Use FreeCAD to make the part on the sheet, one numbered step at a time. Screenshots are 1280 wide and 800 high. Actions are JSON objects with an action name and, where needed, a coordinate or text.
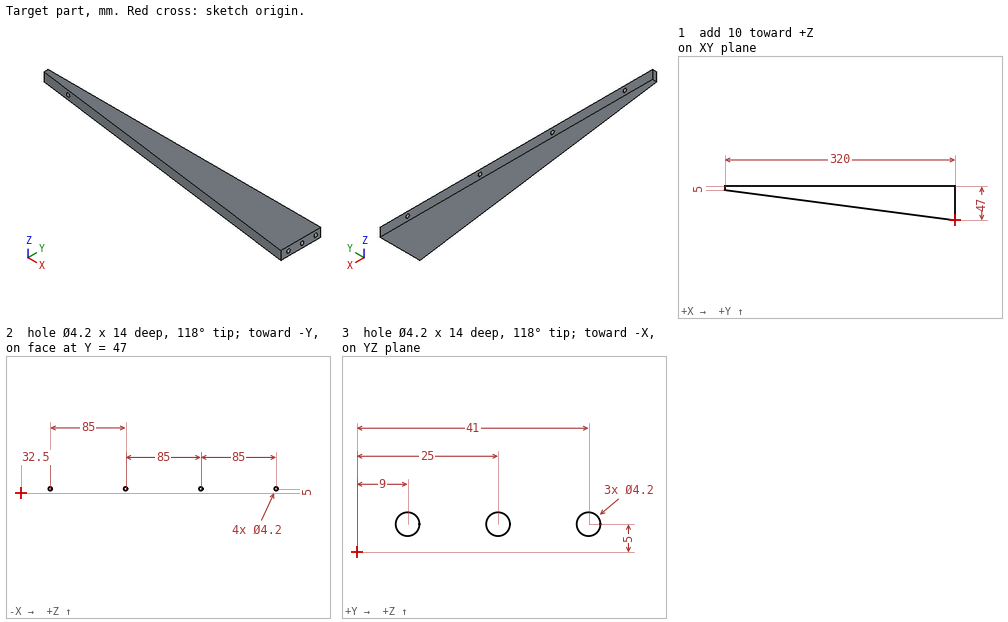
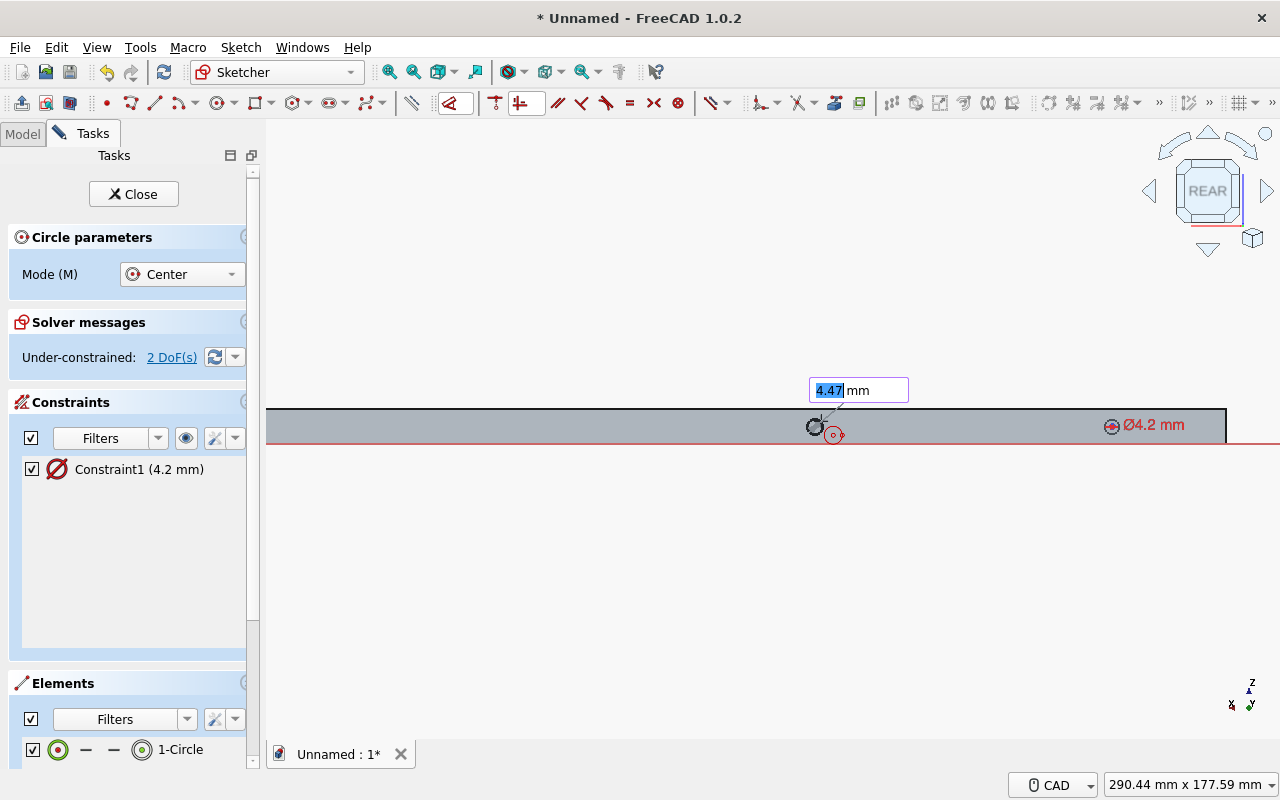
{"action": "type", "text": "4.2"}
{"action": "key", "text": "Return"}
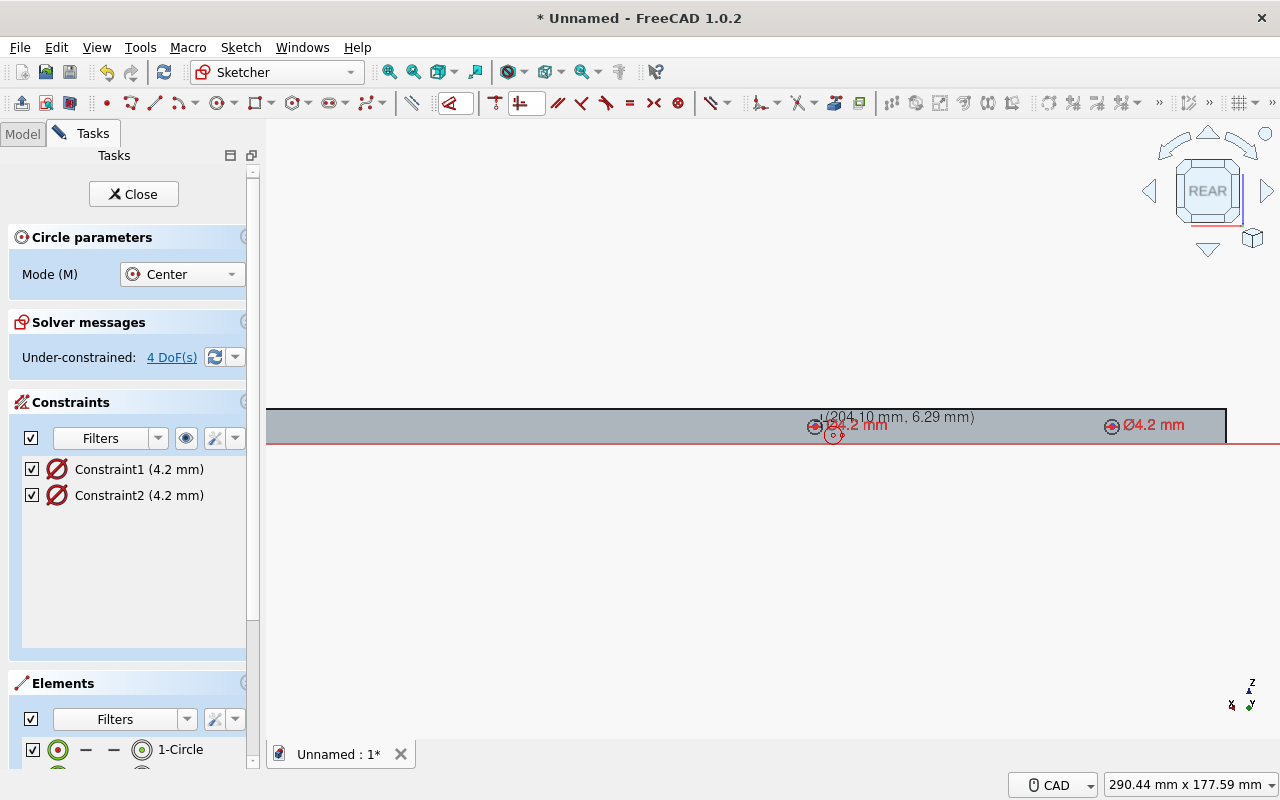
{"action": "scroll", "coordinate": [519, 426], "scroll_direction": "up", "scroll_amount": 6}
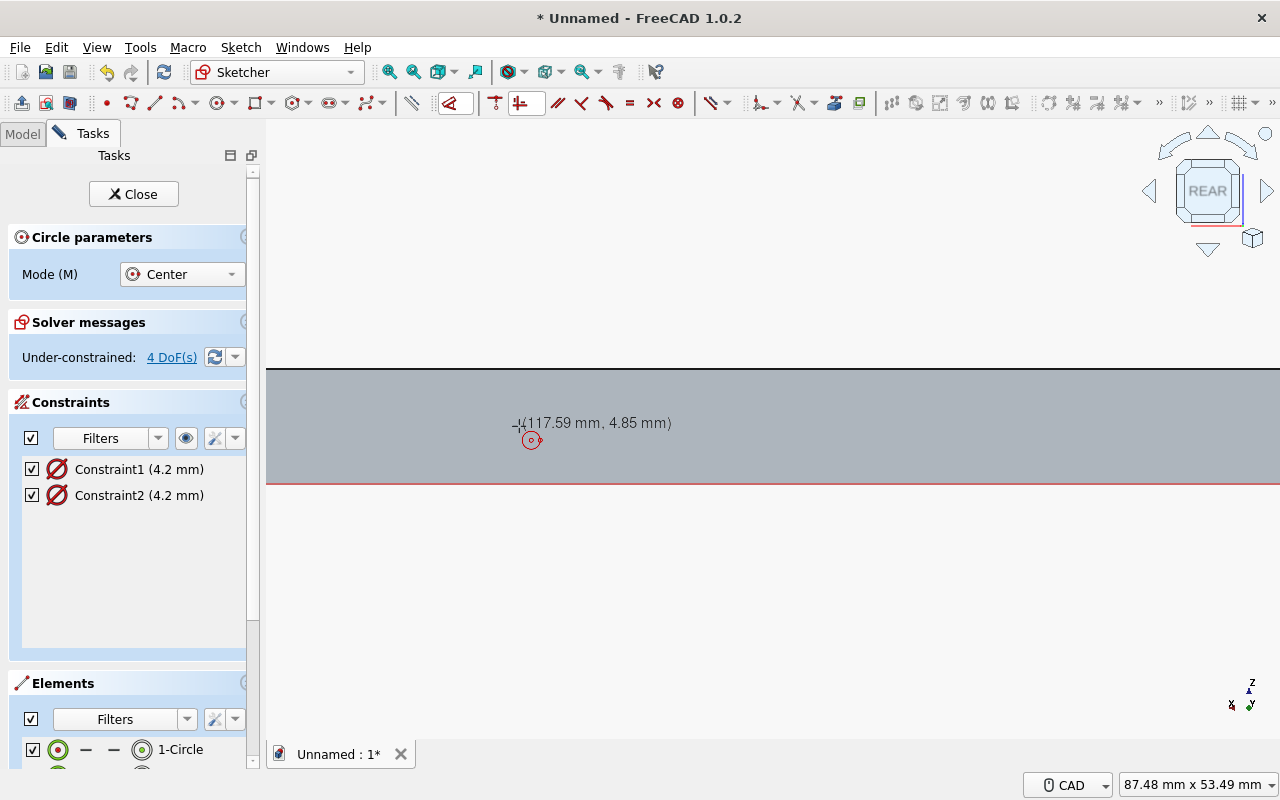
{"action": "scroll", "coordinate": [679, 426], "scroll_direction": "down", "scroll_amount": 9}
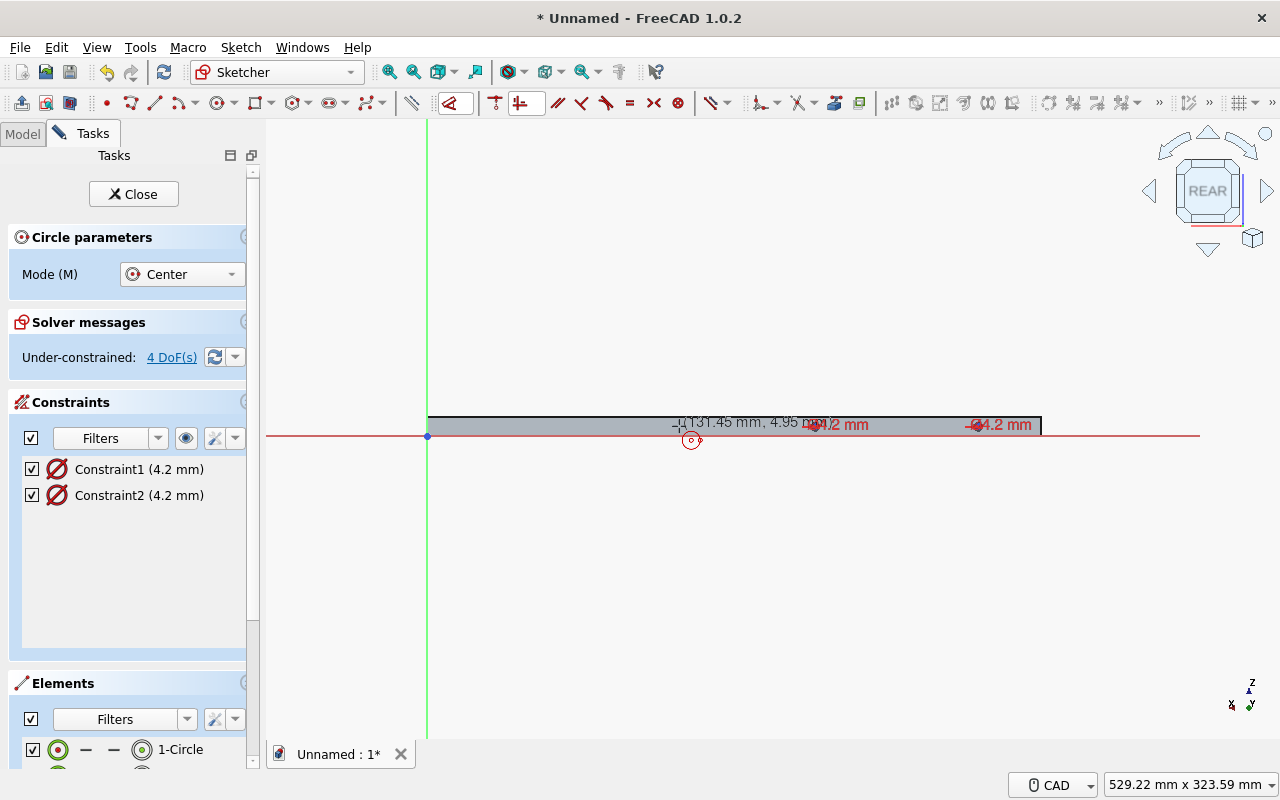
{"action": "scroll", "coordinate": [653, 426], "scroll_direction": "up", "scroll_amount": 3}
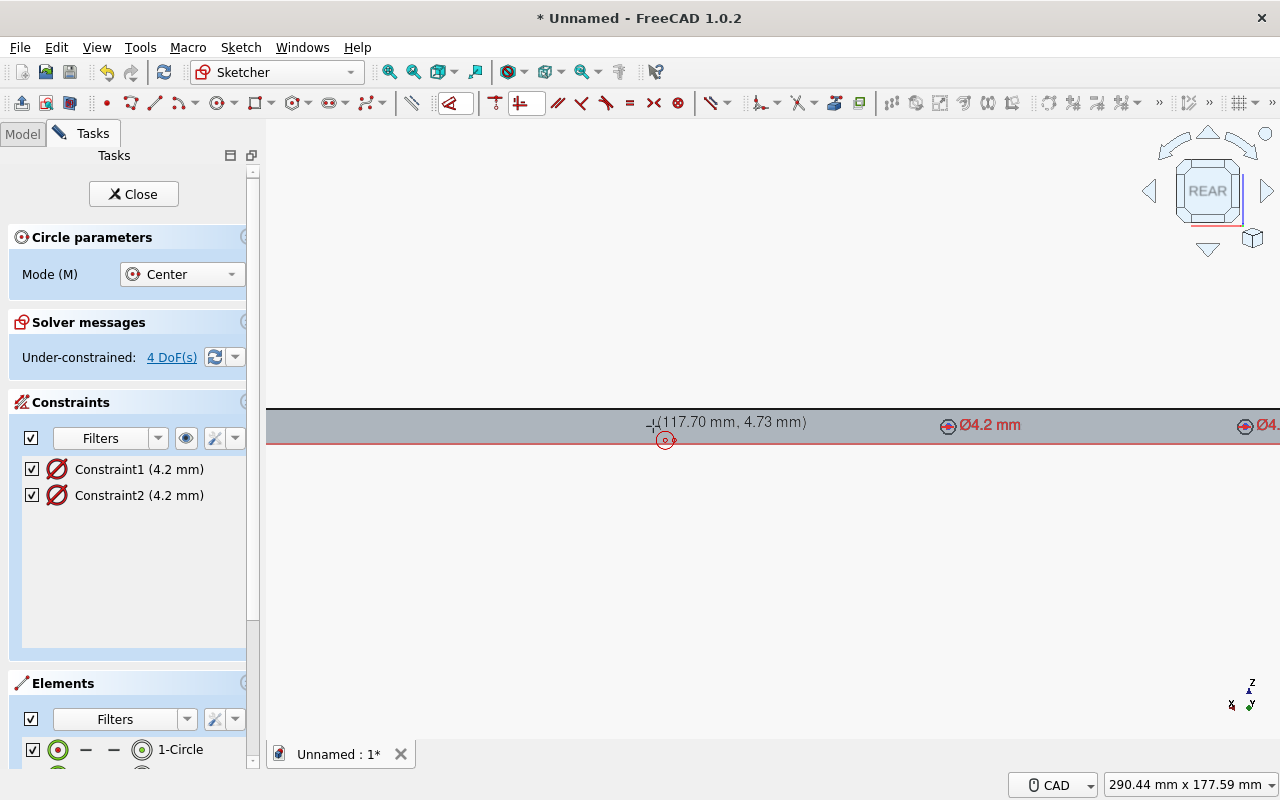
{"action": "left_click", "coordinate": [652, 426]}
{"action": "mouse_move", "coordinate": [657, 421]}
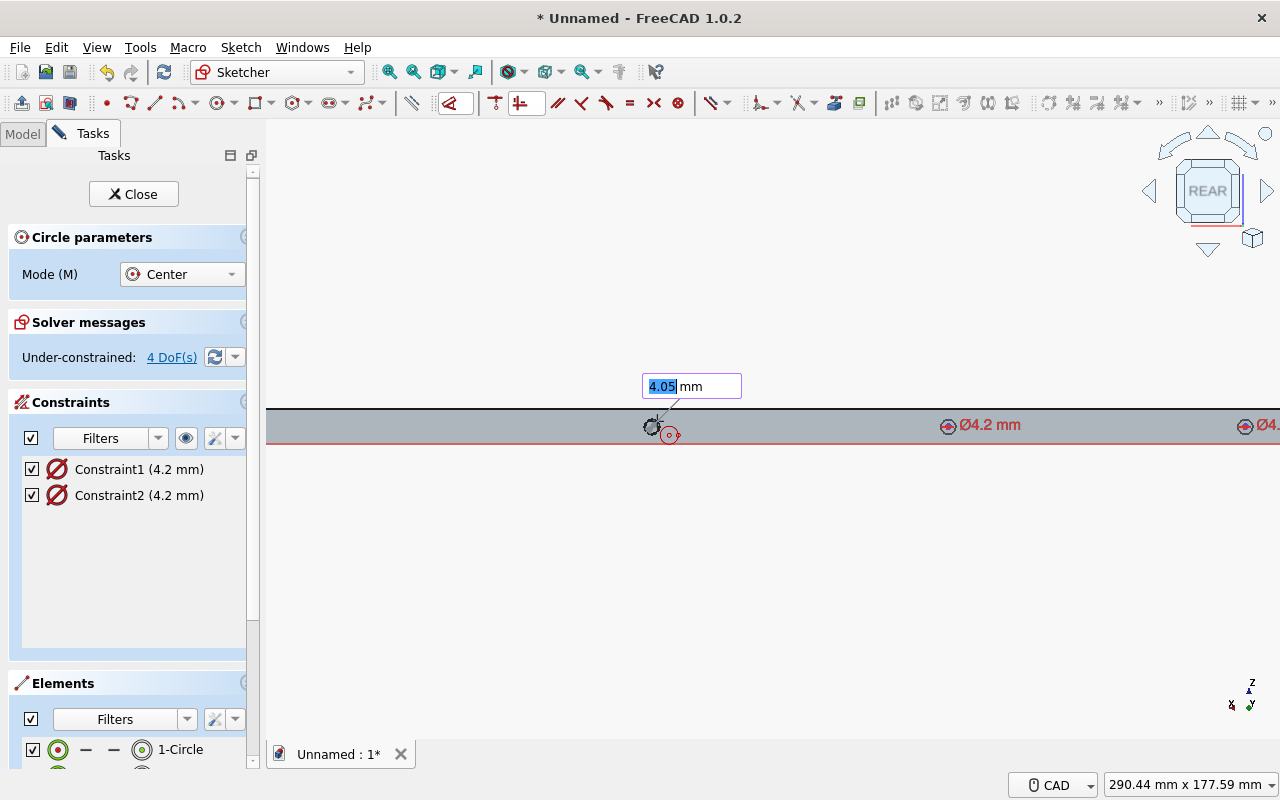
{"action": "type", "text": "4.2"}
{"action": "key", "text": "Return"}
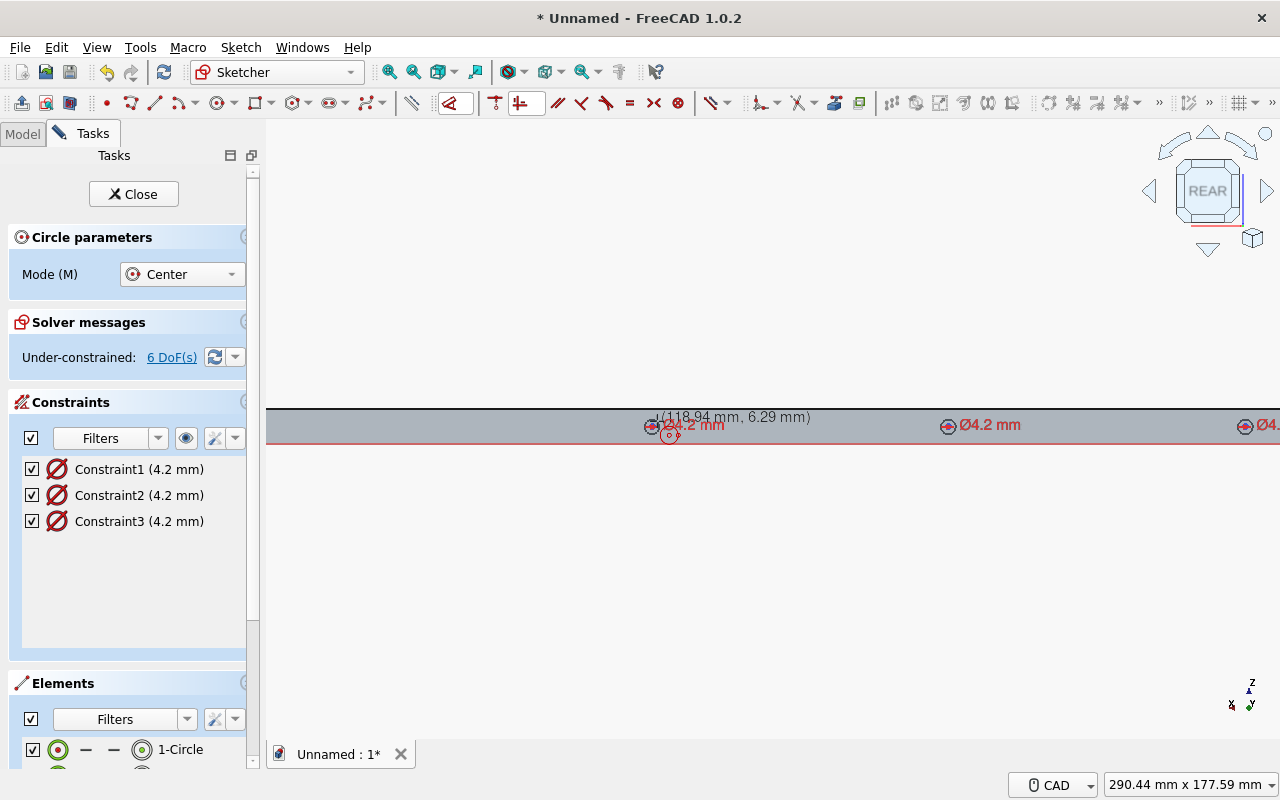
{"action": "scroll", "coordinate": [355, 426], "scroll_direction": "up", "scroll_amount": 6}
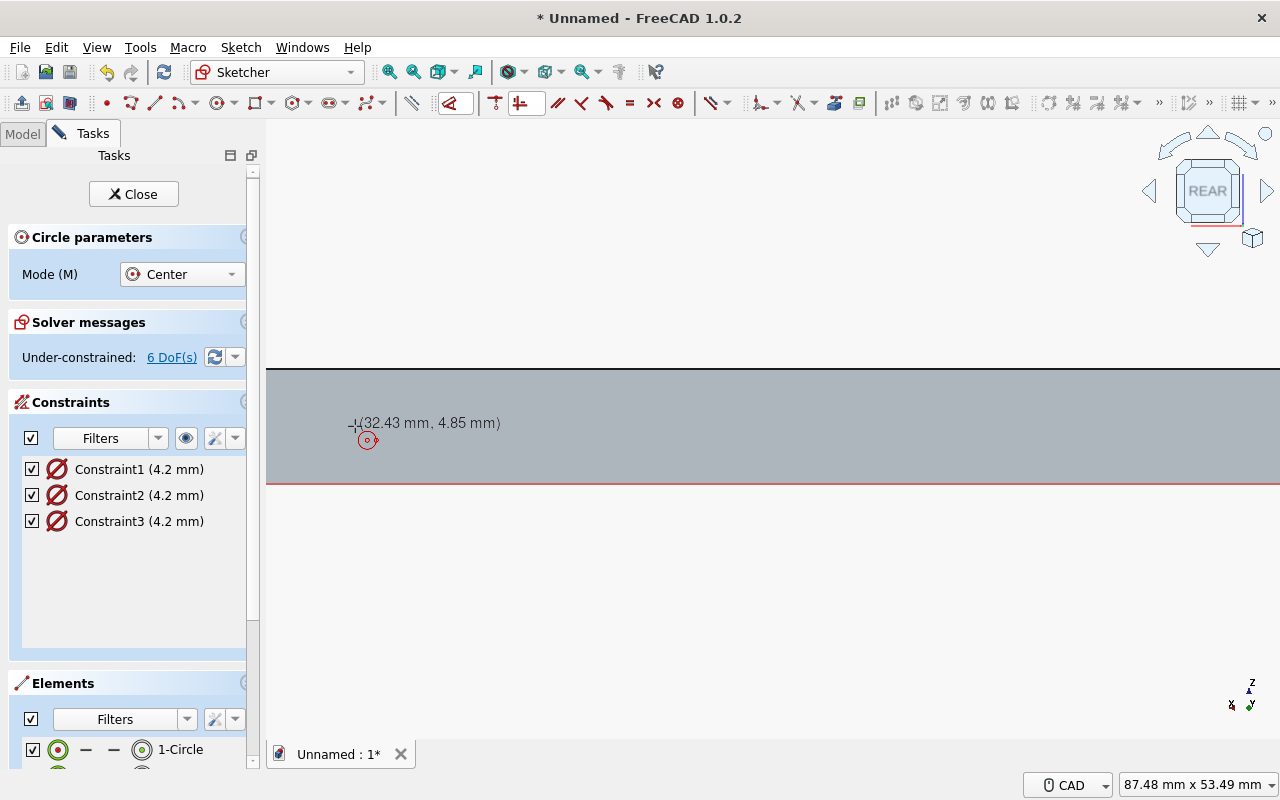
{"action": "scroll", "coordinate": [516, 426], "scroll_direction": "down", "scroll_amount": 9}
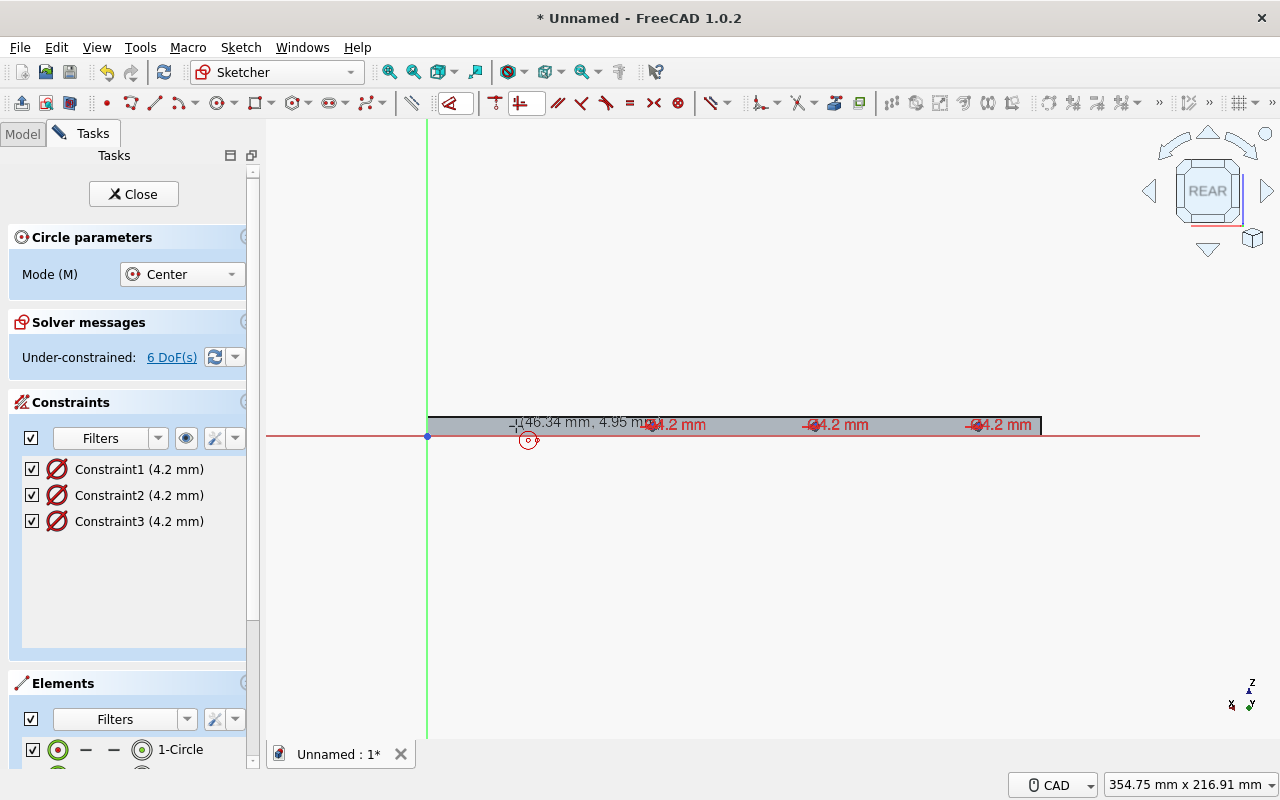
{"action": "scroll", "coordinate": [490, 426], "scroll_direction": "up", "scroll_amount": 3}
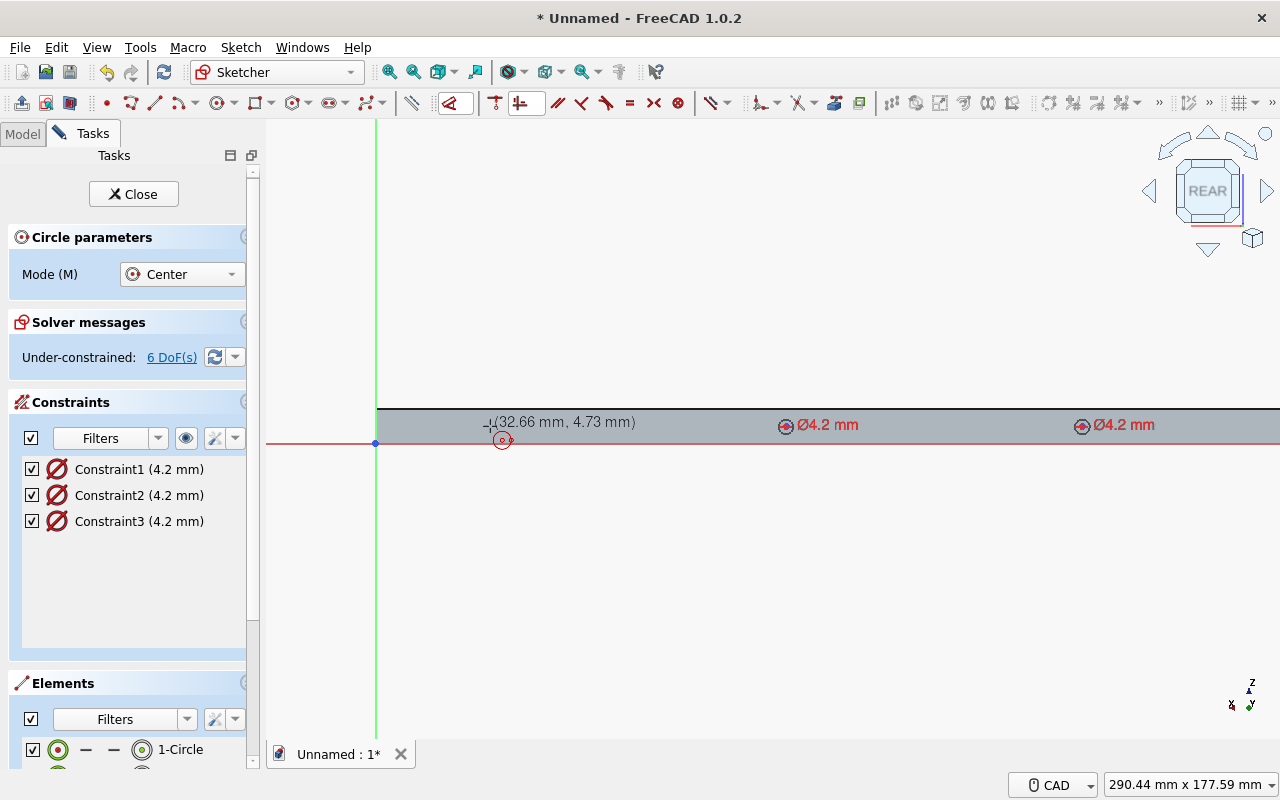
{"action": "left_click", "coordinate": [489, 426]}
{"action": "mouse_move", "coordinate": [494, 421]}